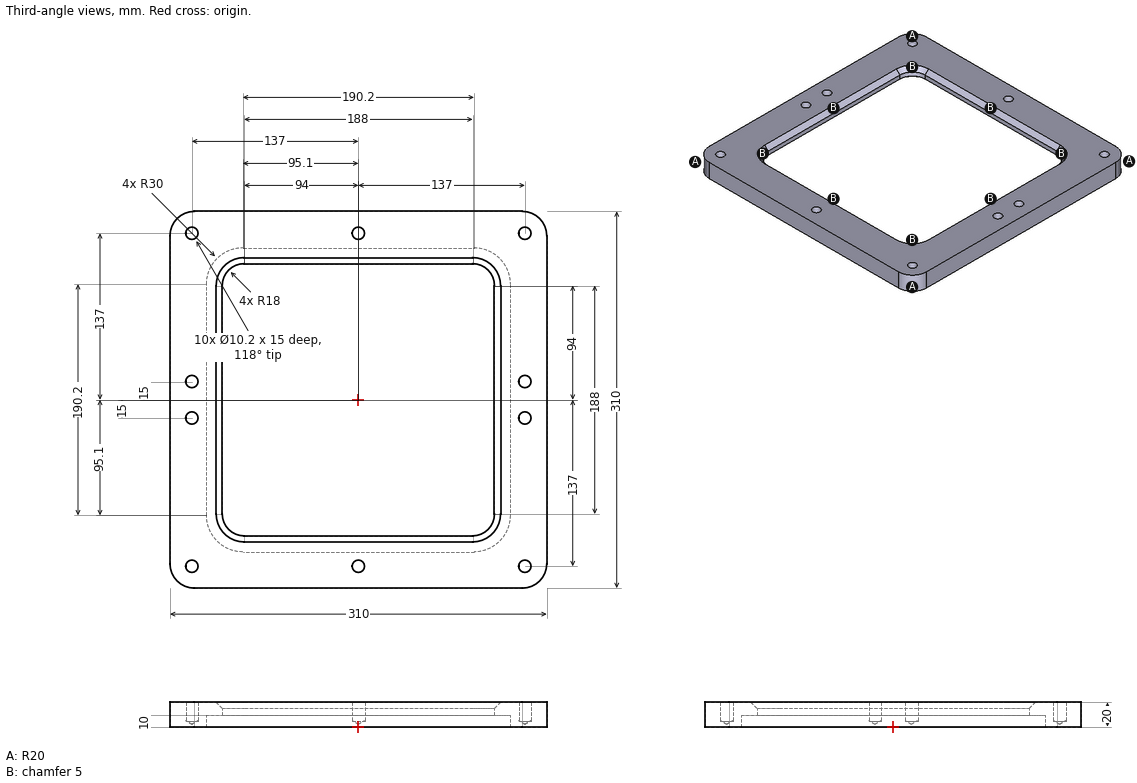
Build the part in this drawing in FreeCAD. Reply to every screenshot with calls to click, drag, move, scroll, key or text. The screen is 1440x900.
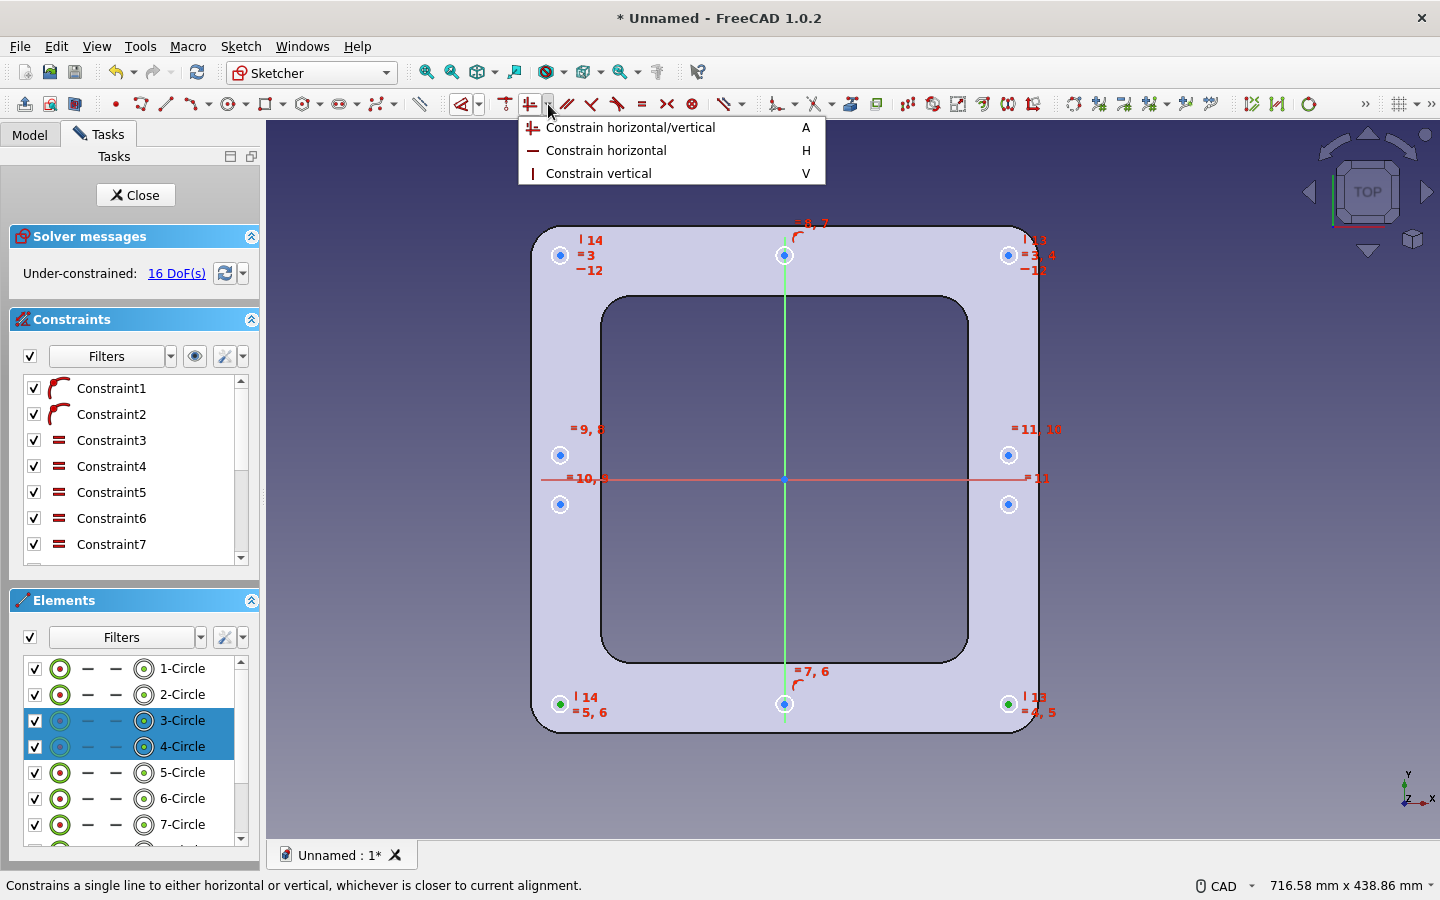
click(672, 150)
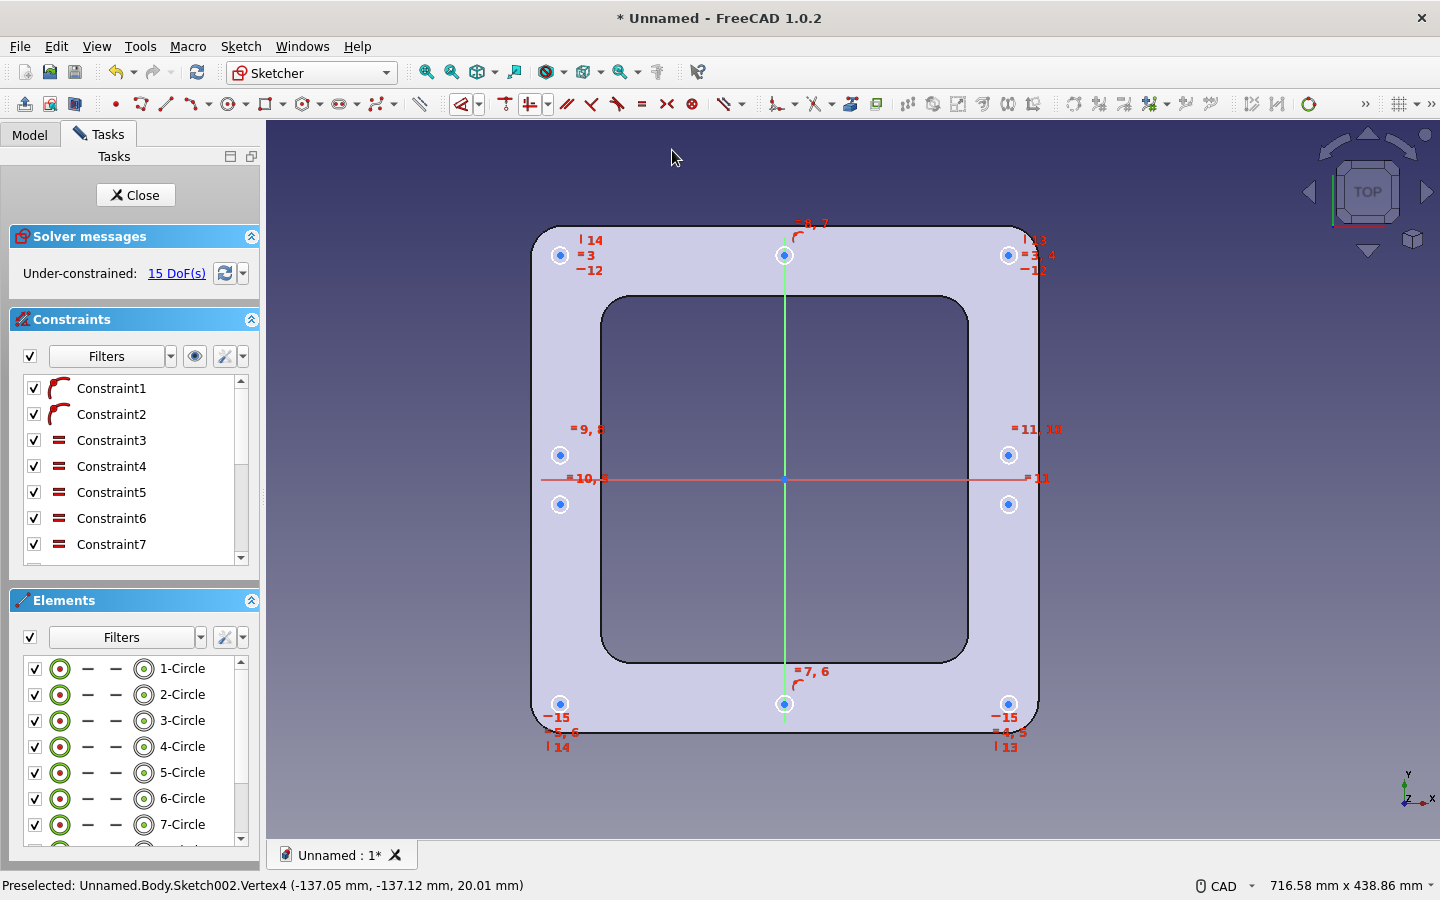
click(1009, 704)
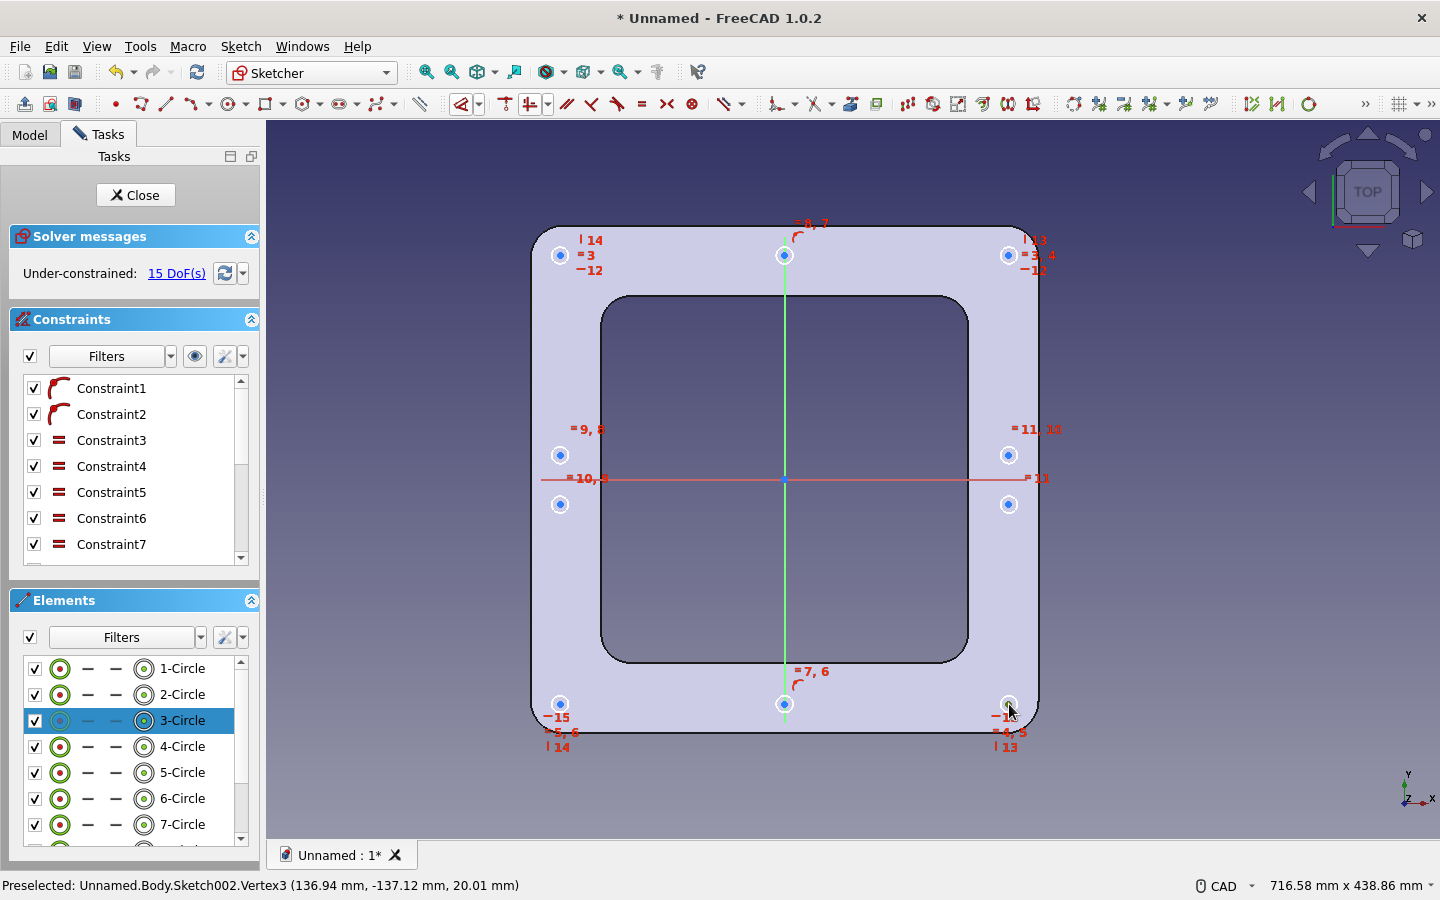
click(785, 704)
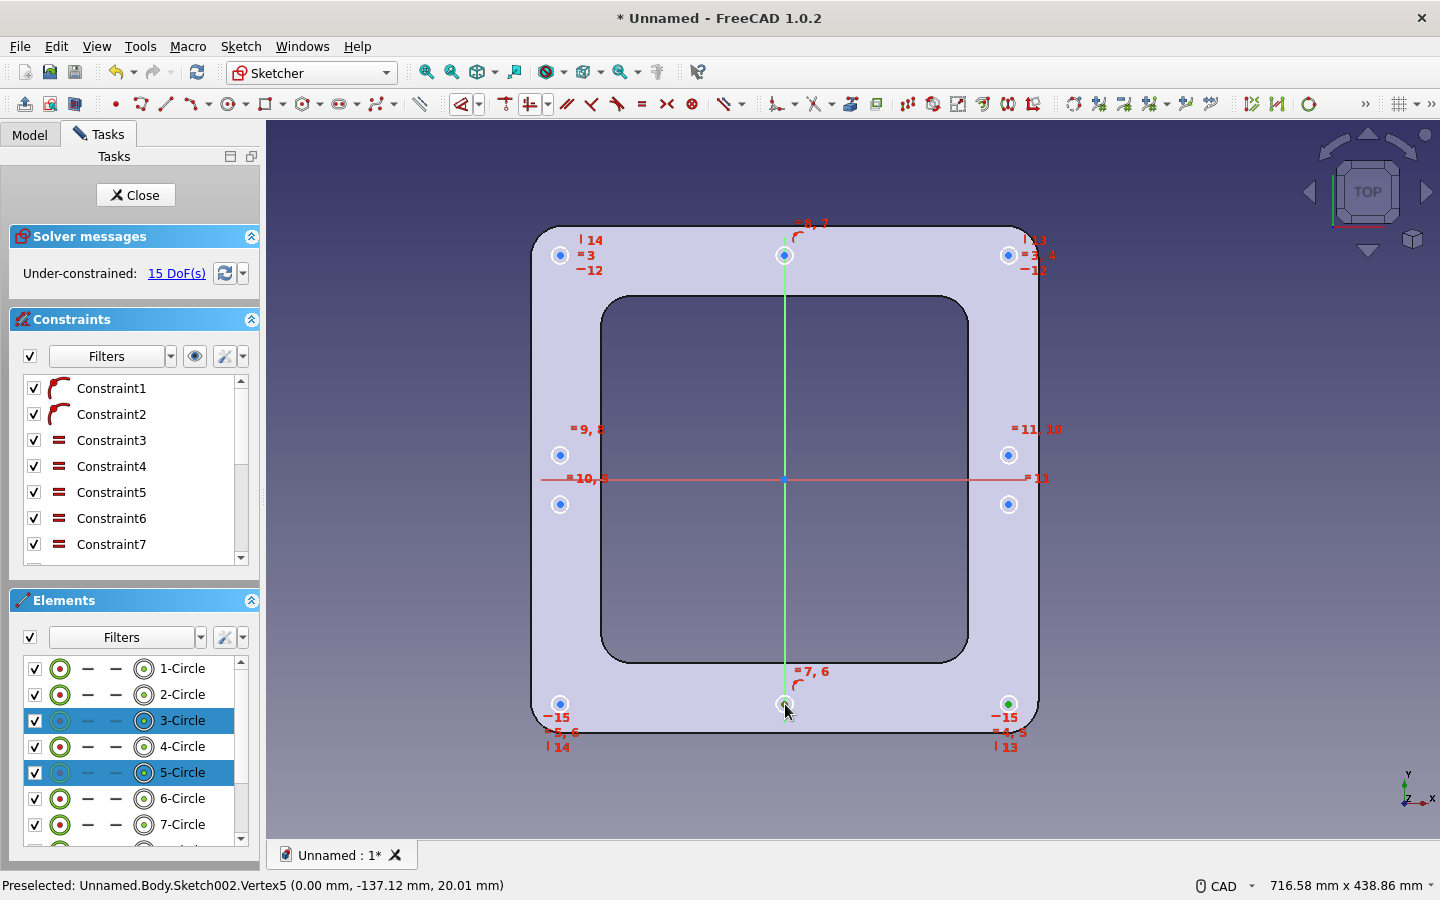
key(h)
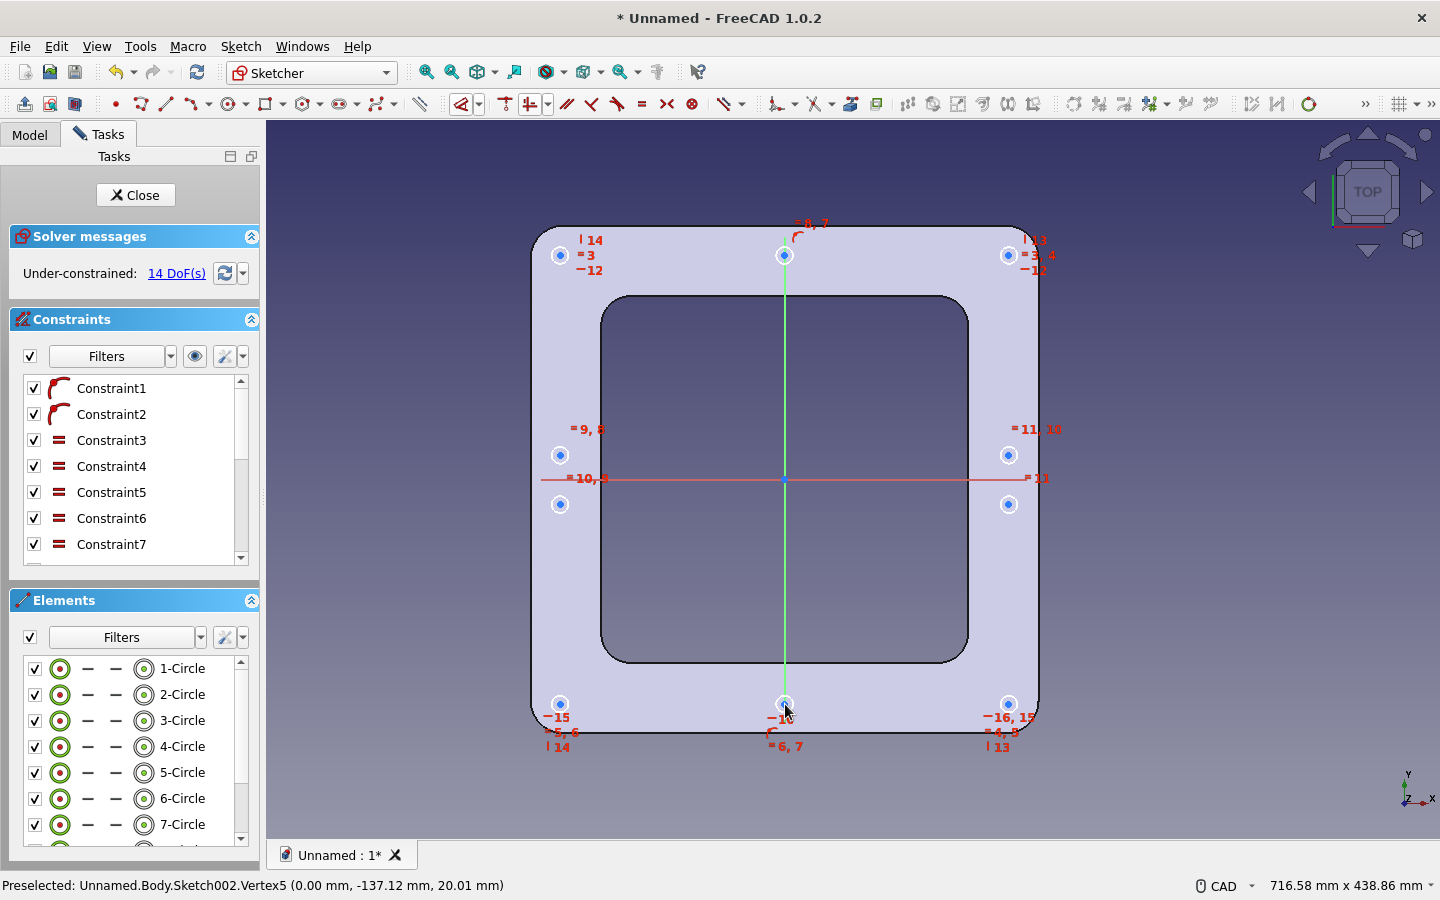
click(560, 255)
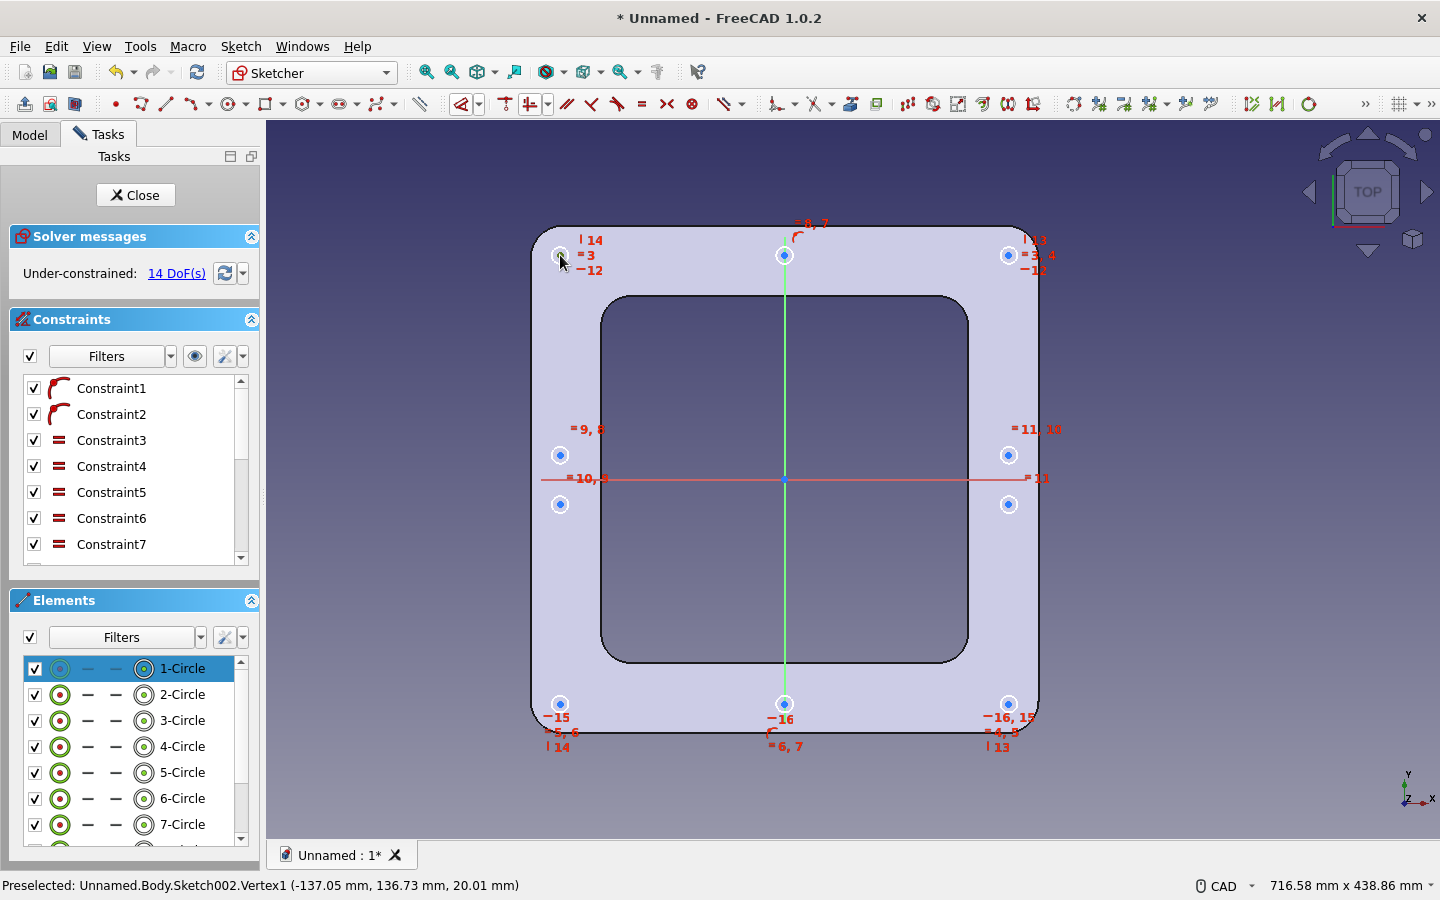
click(785, 255)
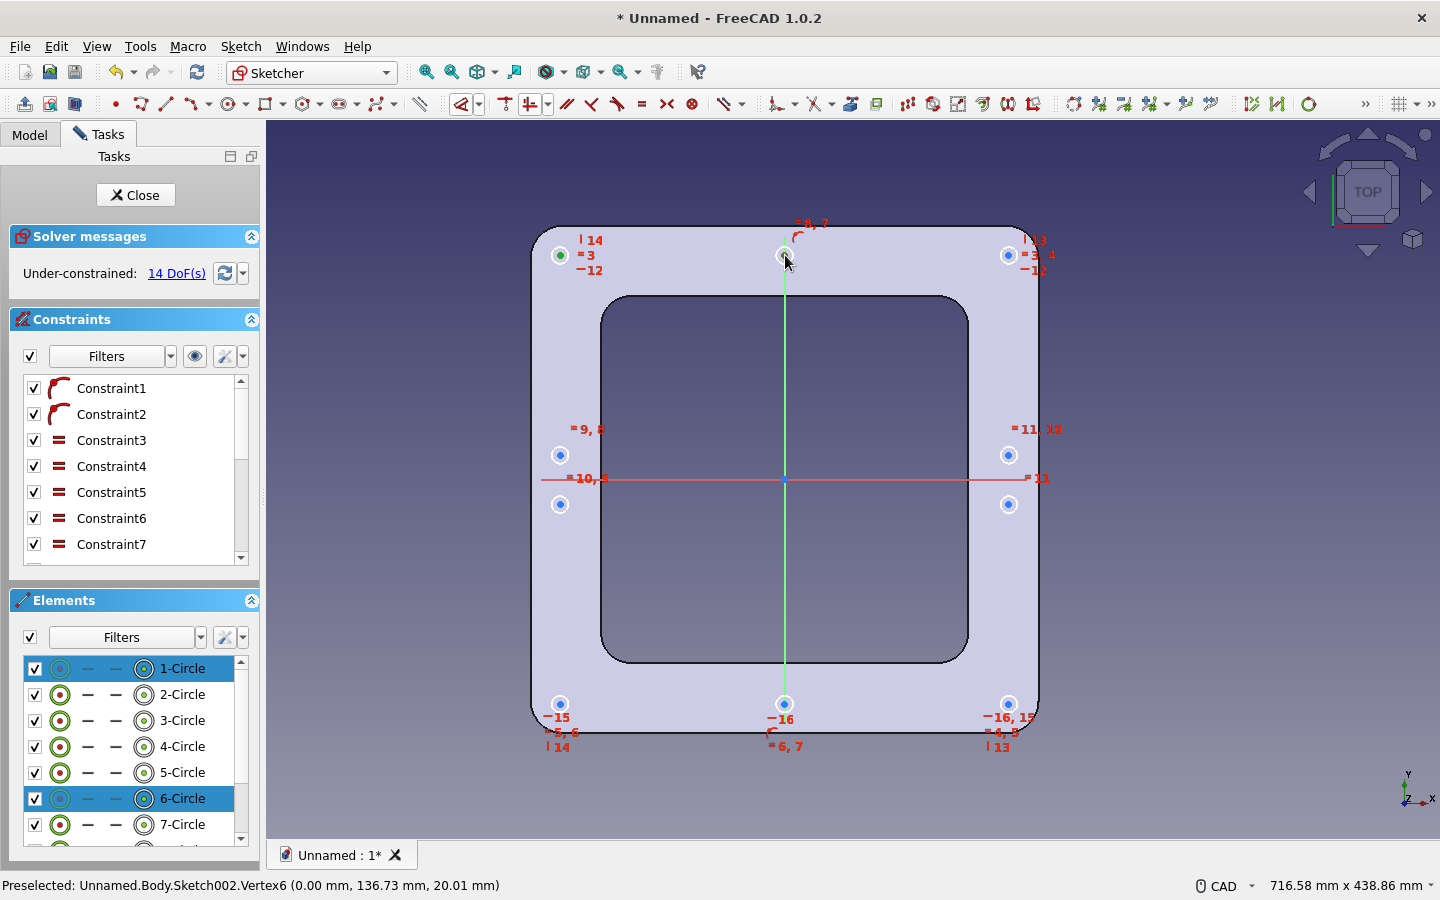
key(h)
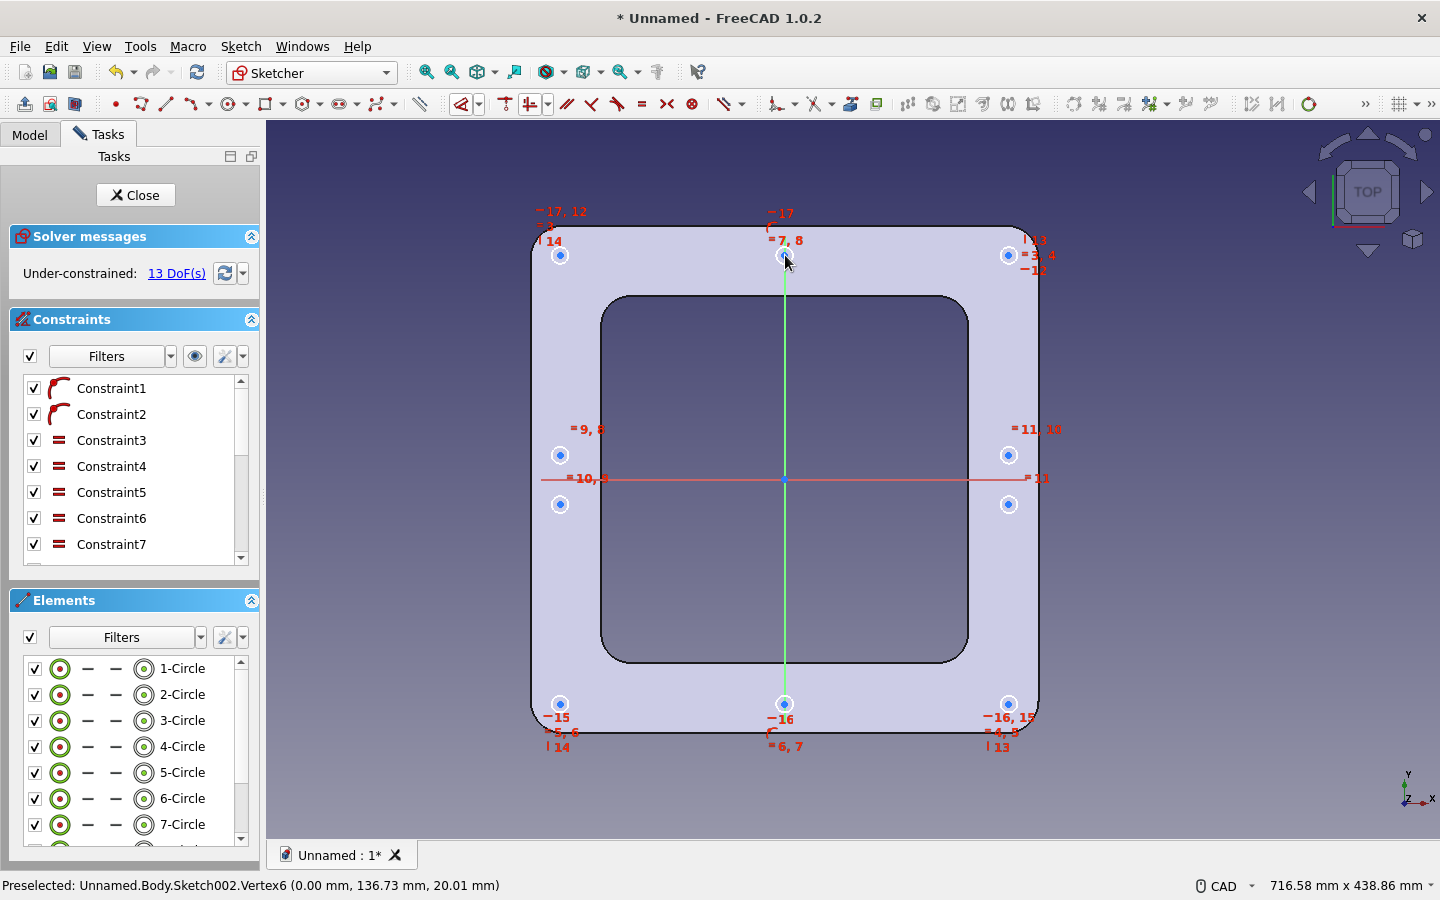
click(560, 255)